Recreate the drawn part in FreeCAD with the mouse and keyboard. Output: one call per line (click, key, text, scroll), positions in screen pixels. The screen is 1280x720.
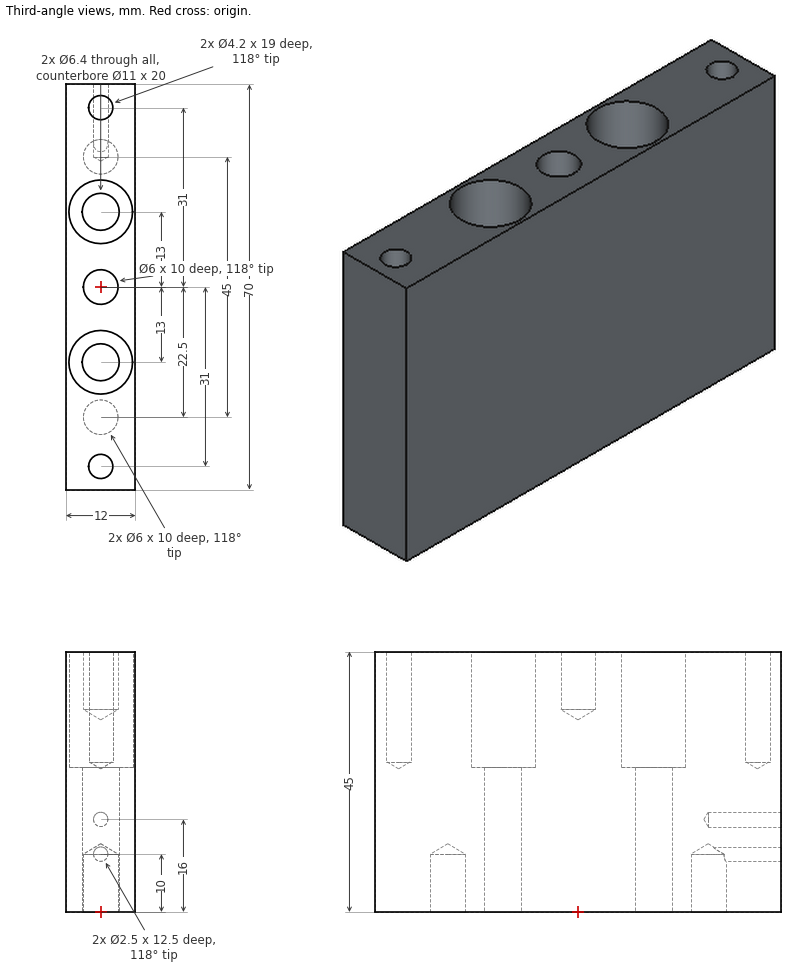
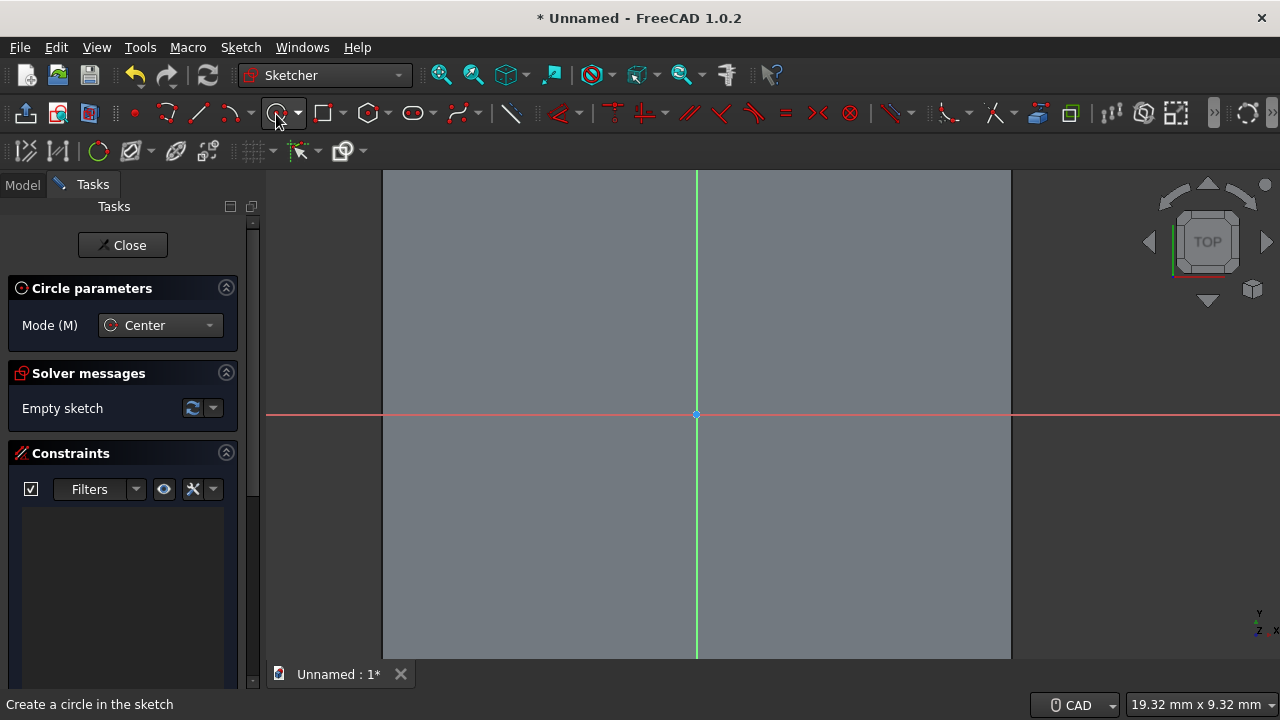
click(697, 414)
move(808, 303)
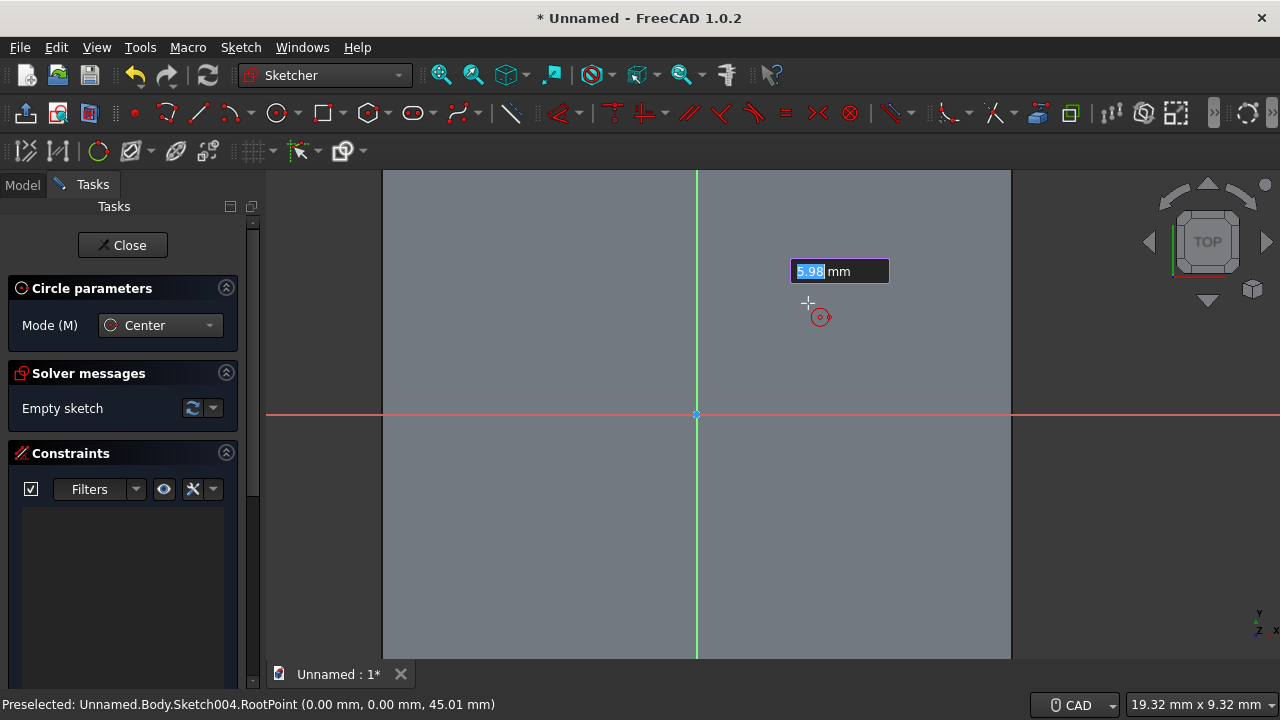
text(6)
key(Return)
key(Escape)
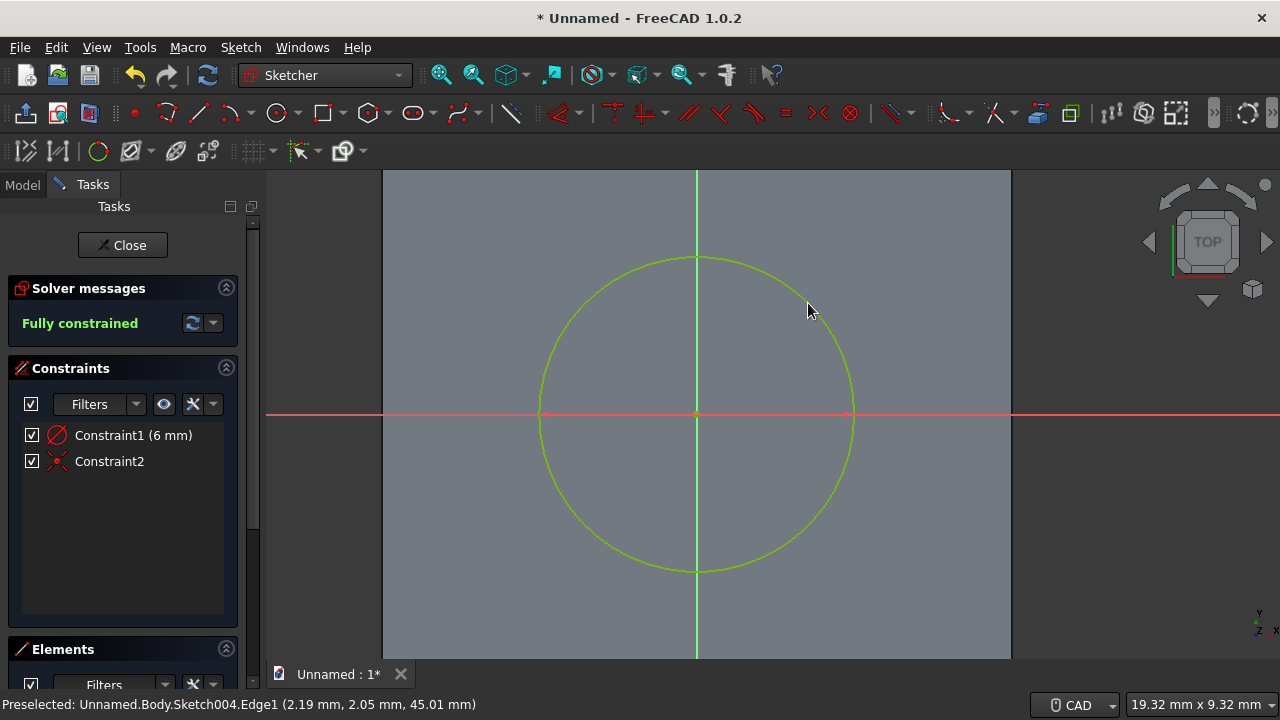
click(123, 245)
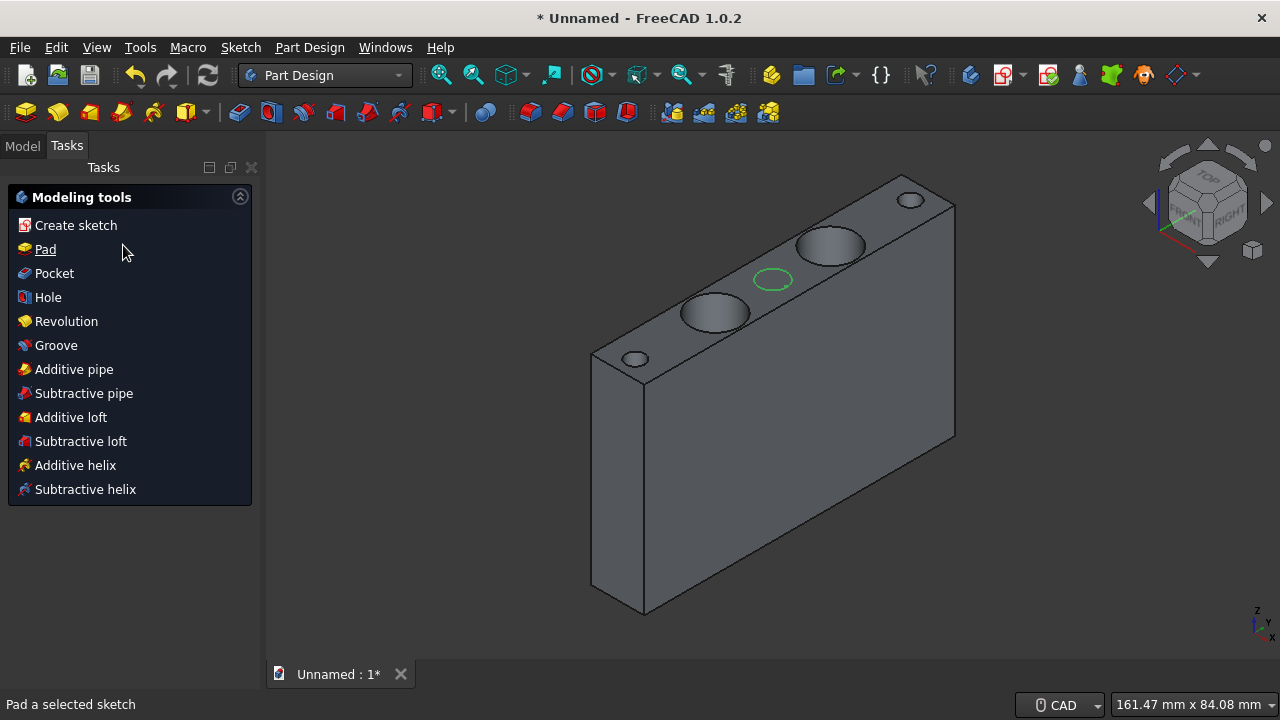
click(272, 112)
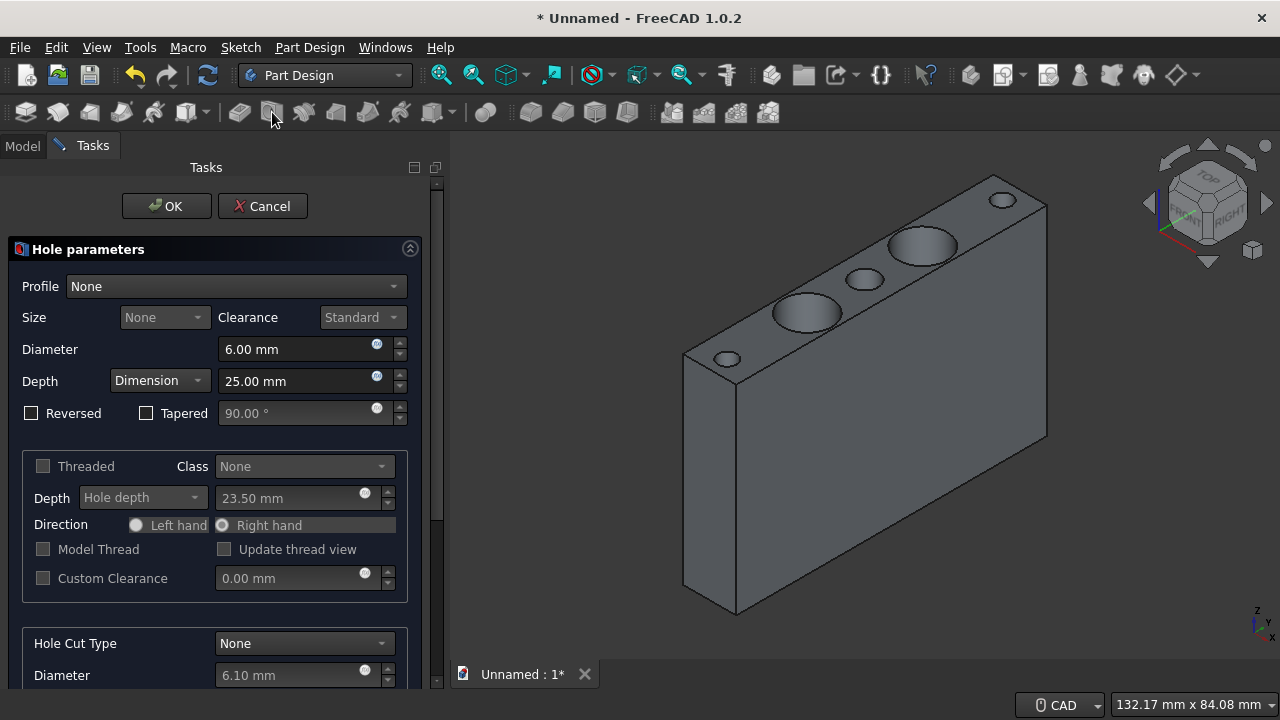
triple_click(305, 349)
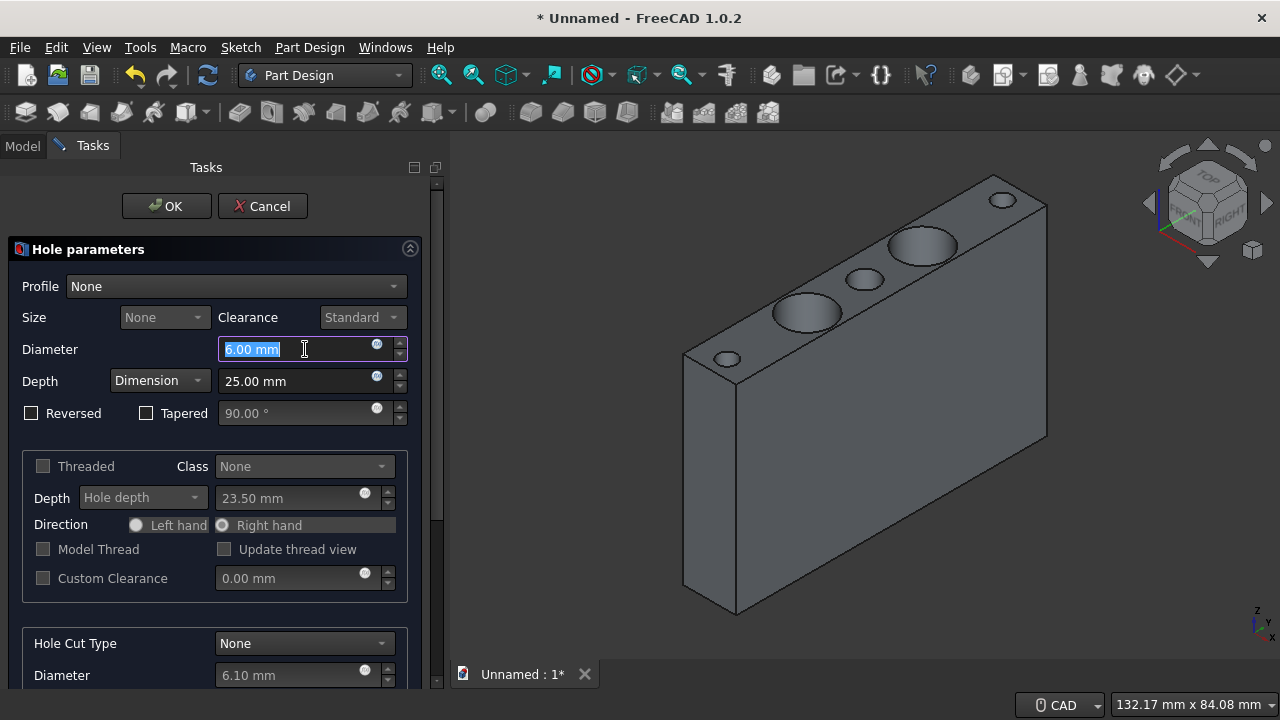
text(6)
key(Tab)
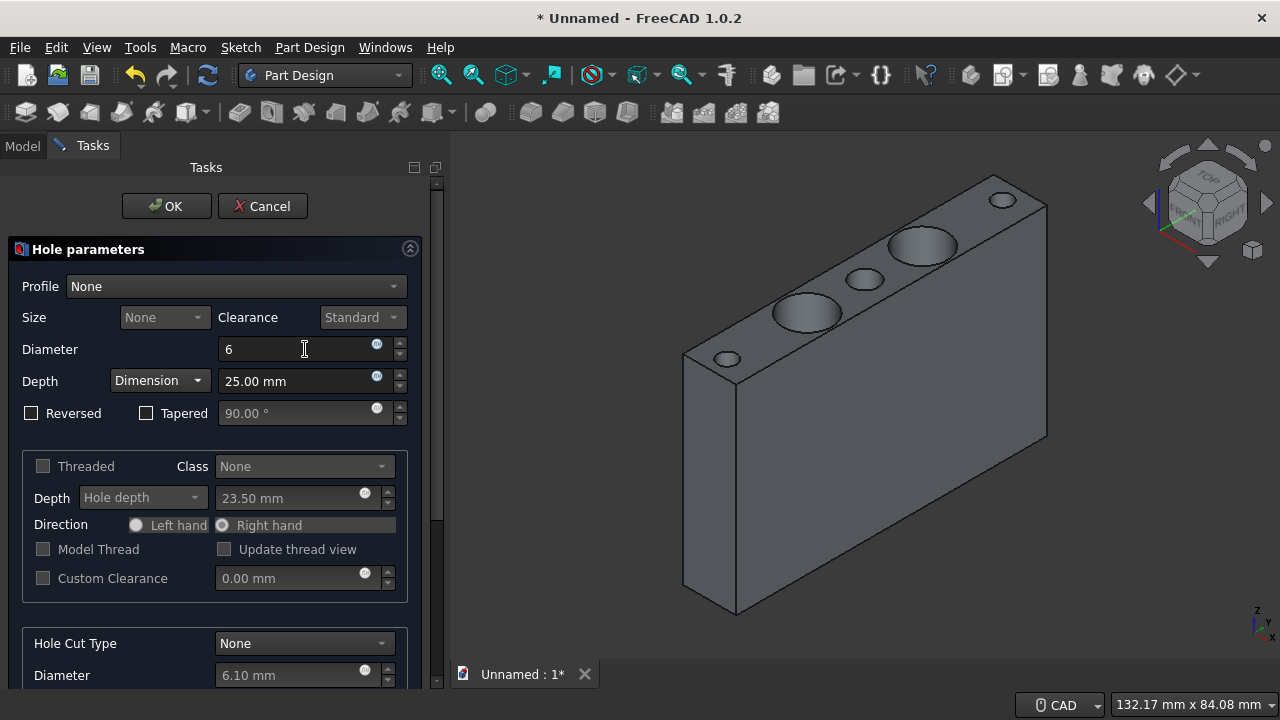
triple_click(305, 381)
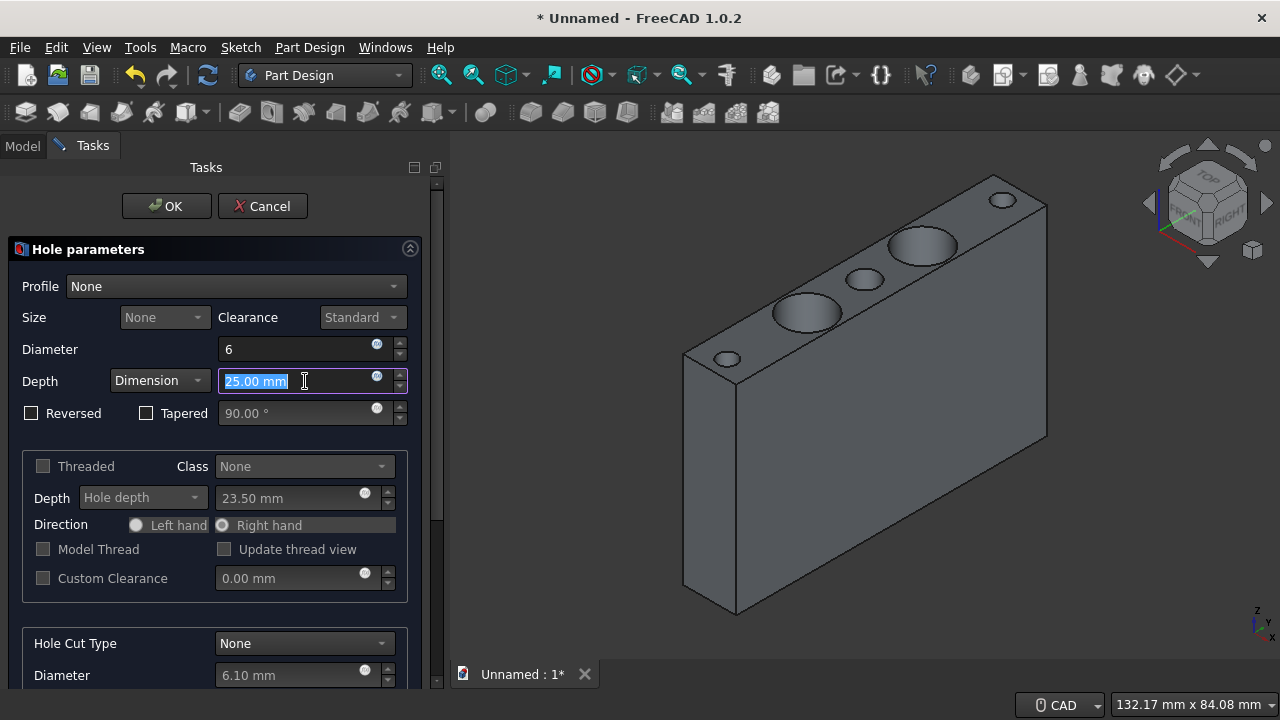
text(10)
key(Tab)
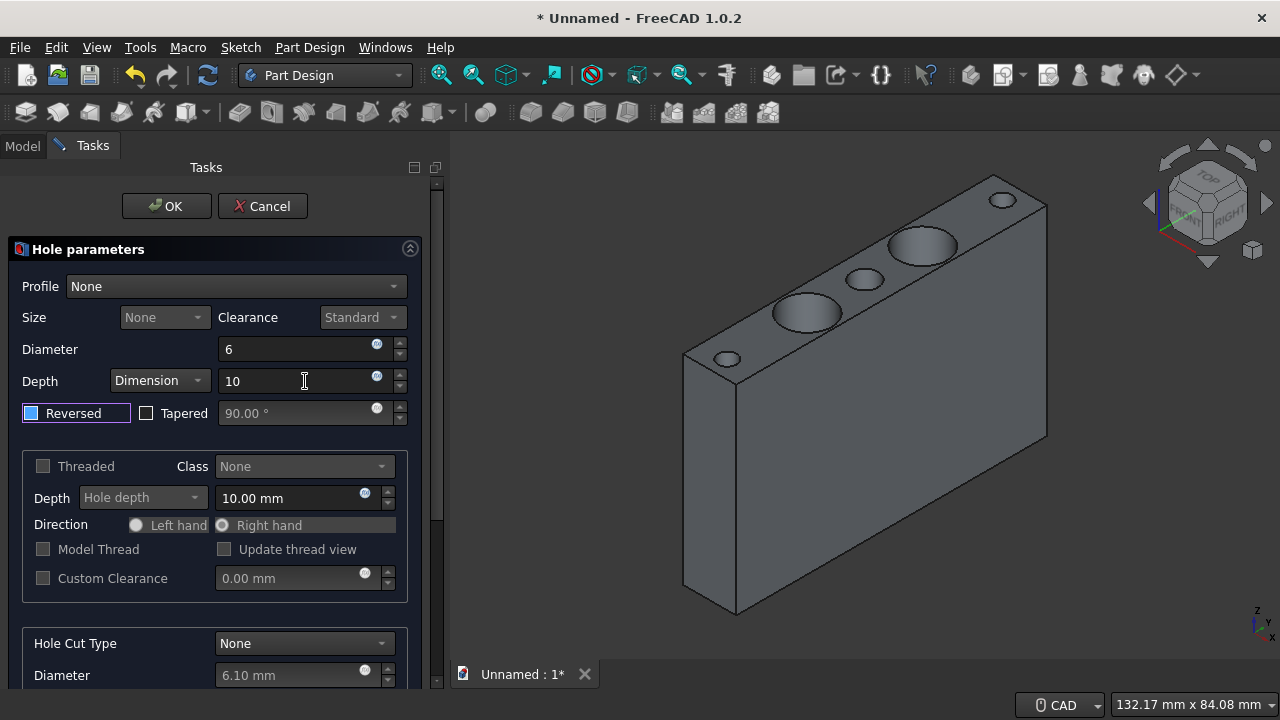
click(167, 206)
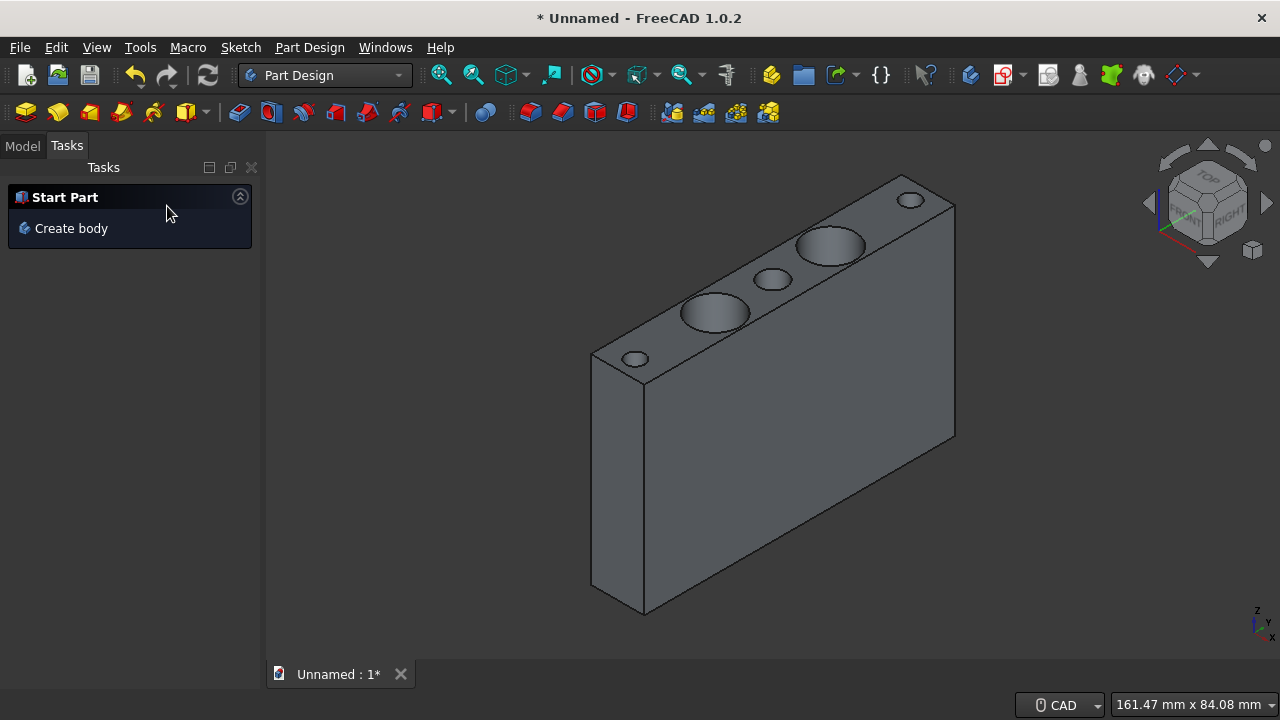
click(1004, 76)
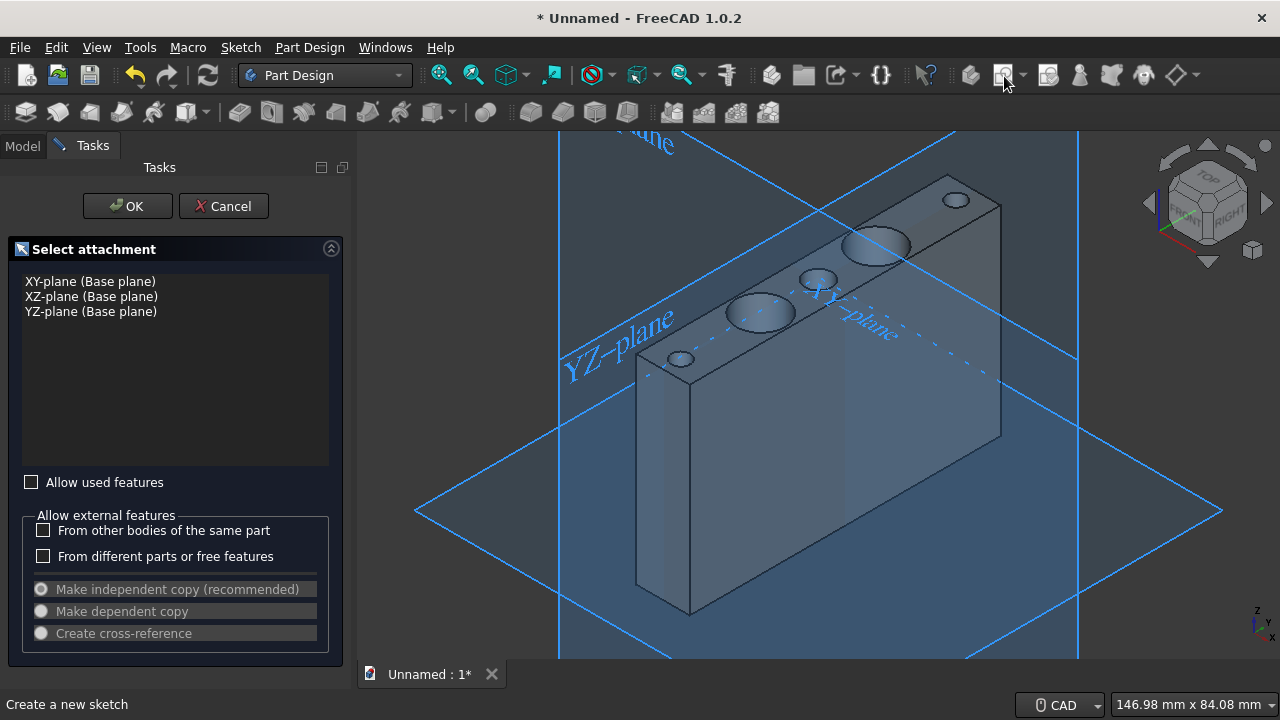
click(82, 282)